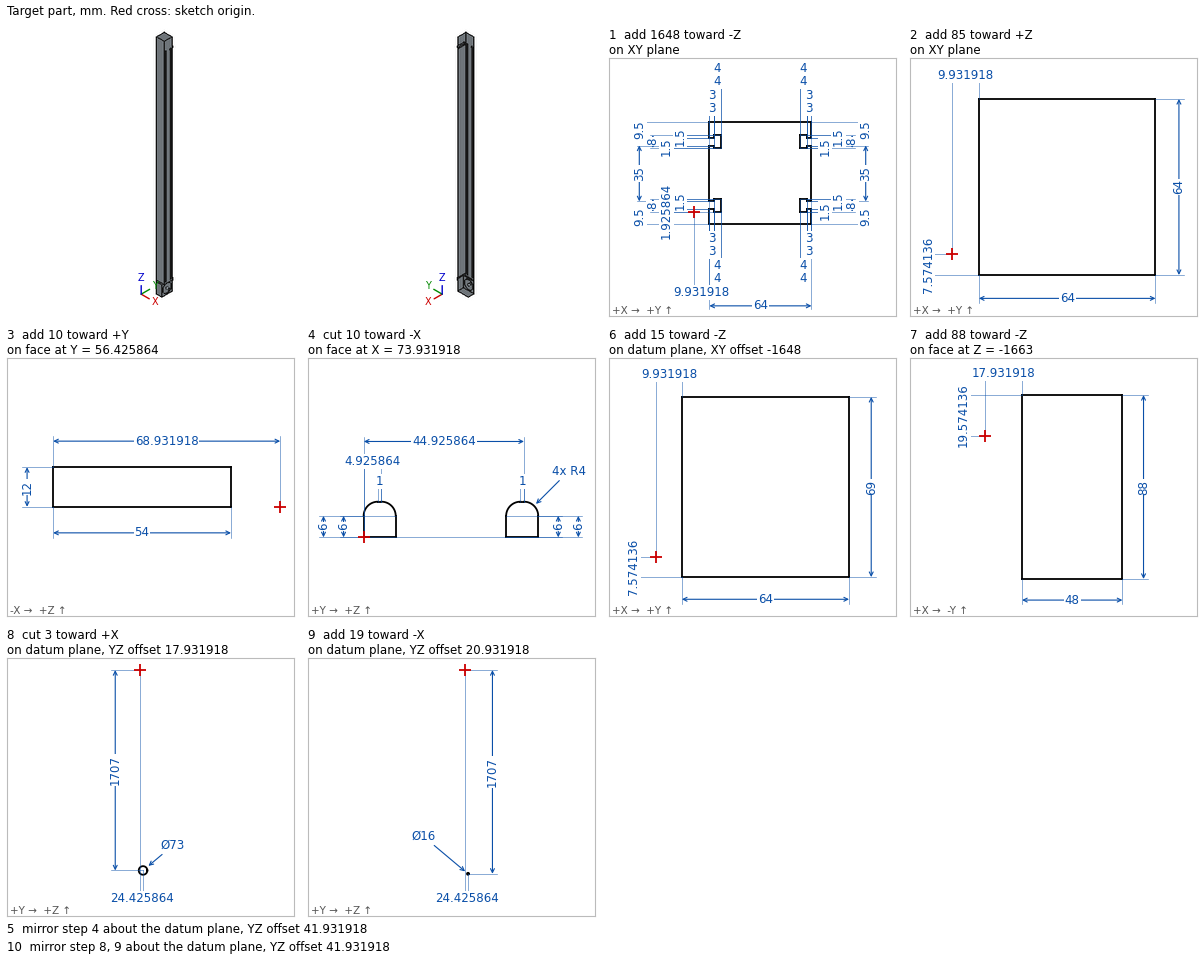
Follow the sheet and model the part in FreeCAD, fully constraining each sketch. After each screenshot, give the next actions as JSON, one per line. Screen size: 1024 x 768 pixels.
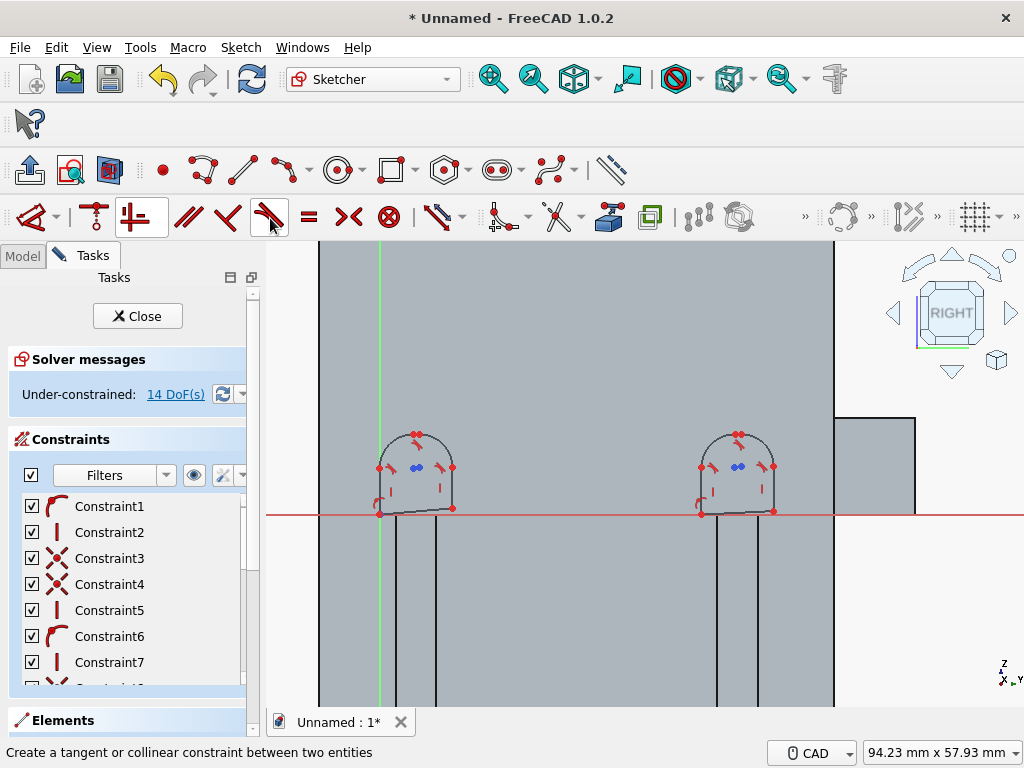
{"action": "left_click", "coordinate": [723, 514]}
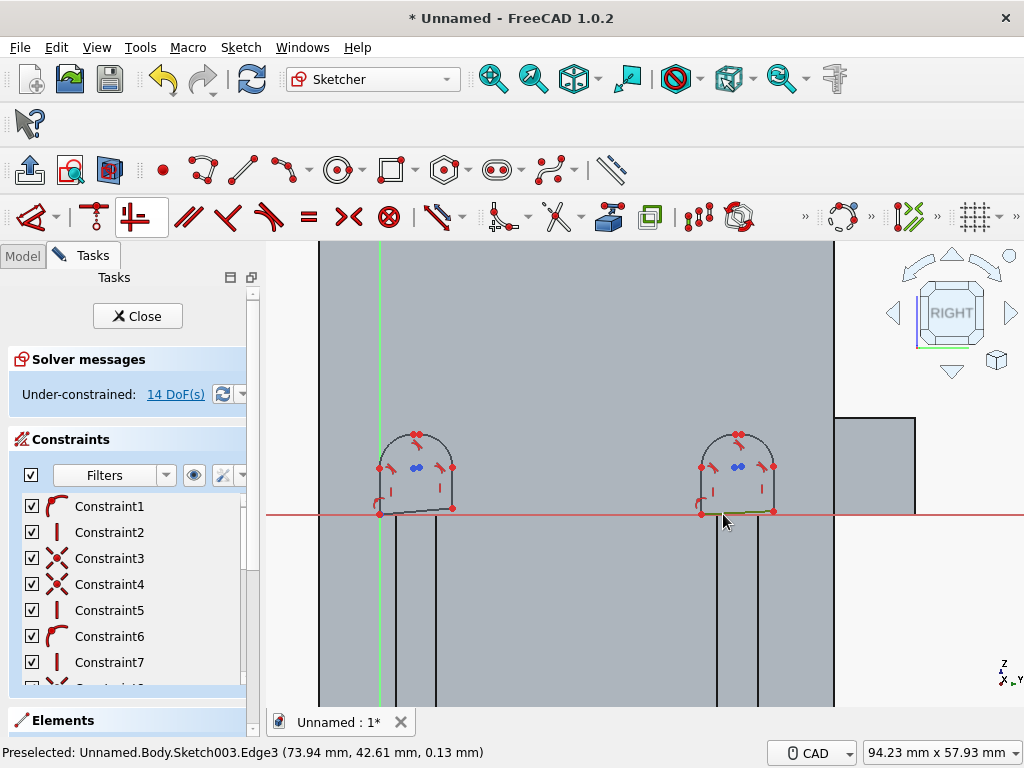
{"action": "left_click", "coordinate": [162, 218]}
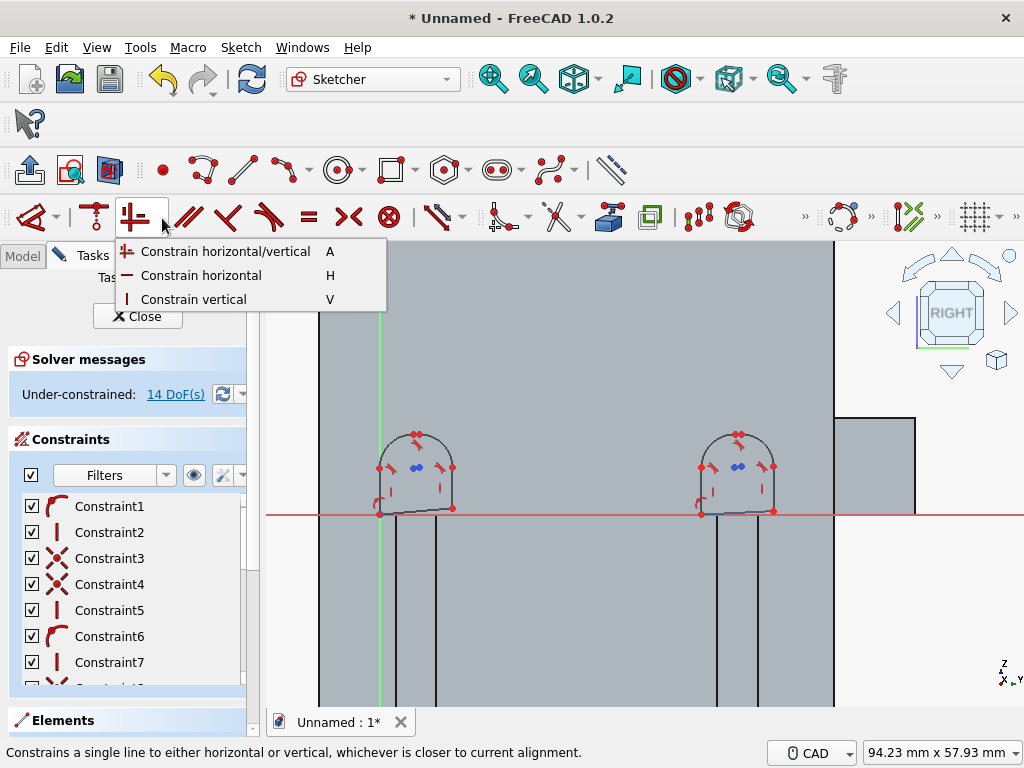
{"action": "left_click", "coordinate": [251, 275]}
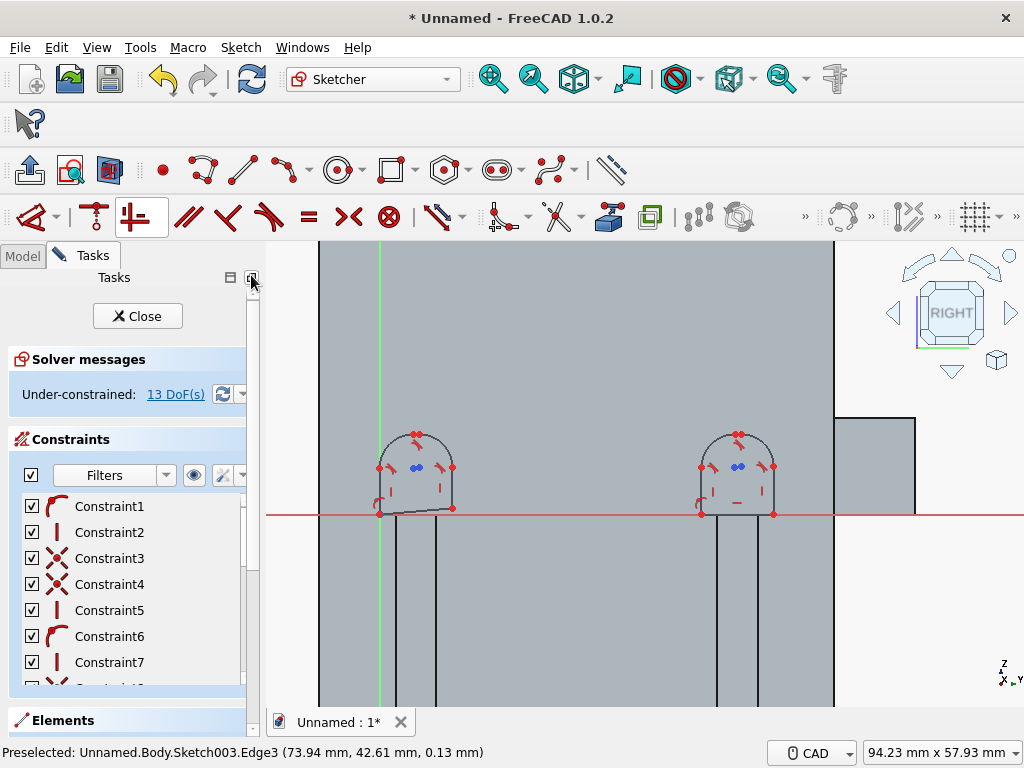
{"action": "left_click", "coordinate": [402, 513]}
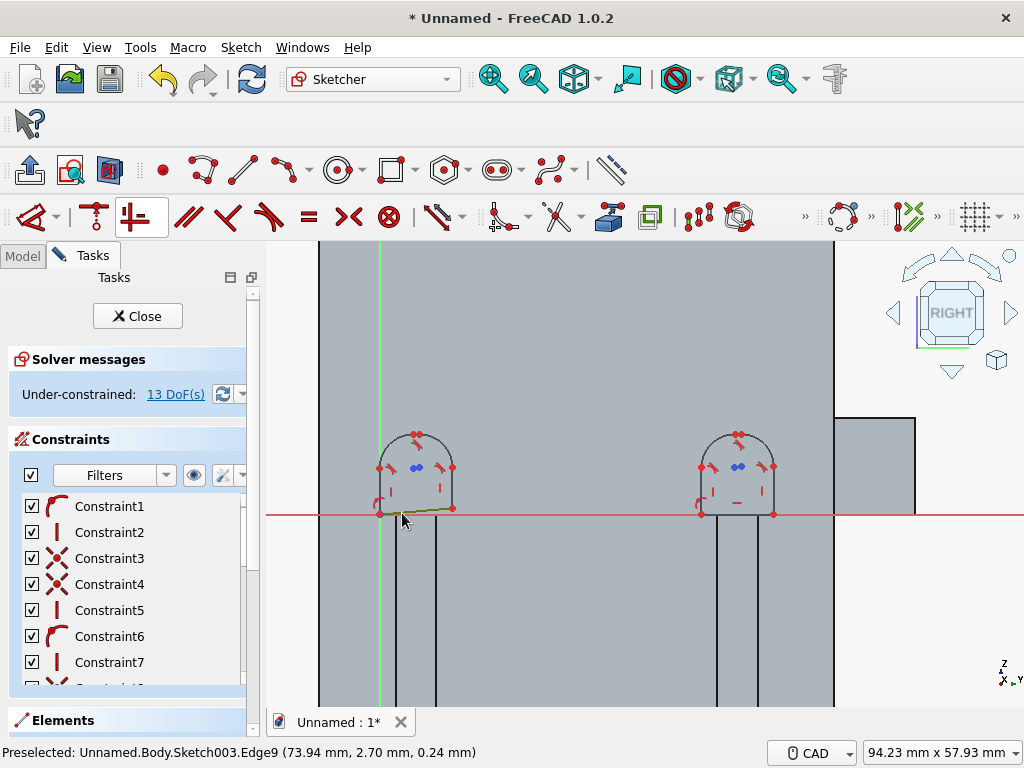
{"action": "key", "text": "h"}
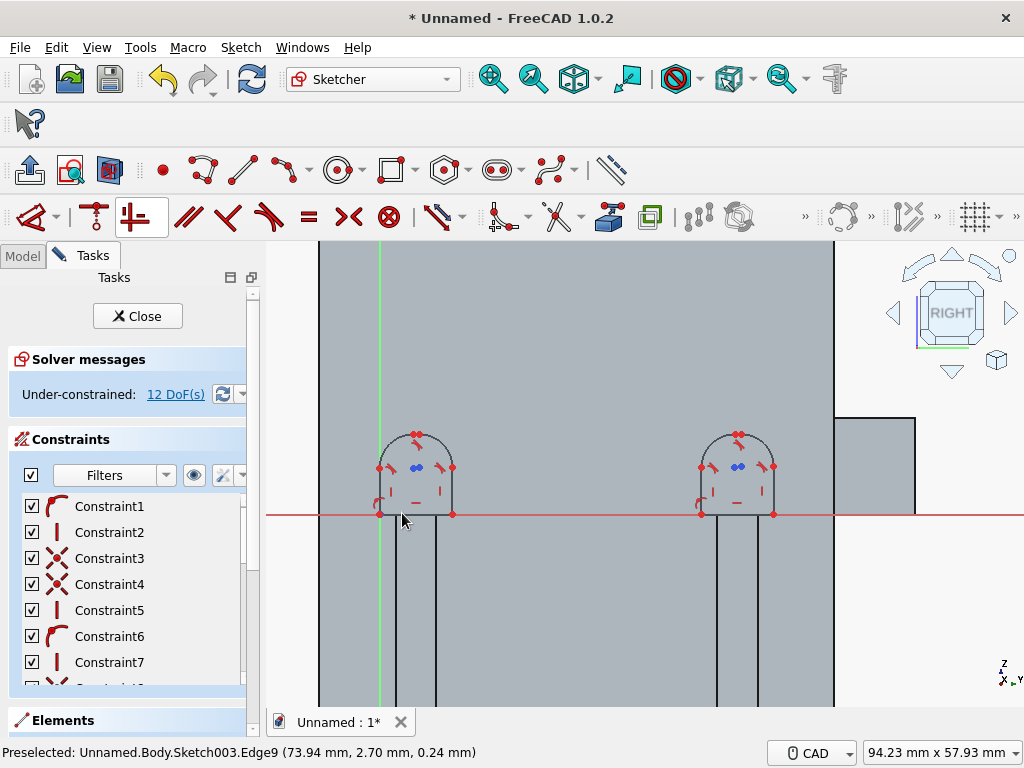
{"action": "left_click", "coordinate": [720, 438]}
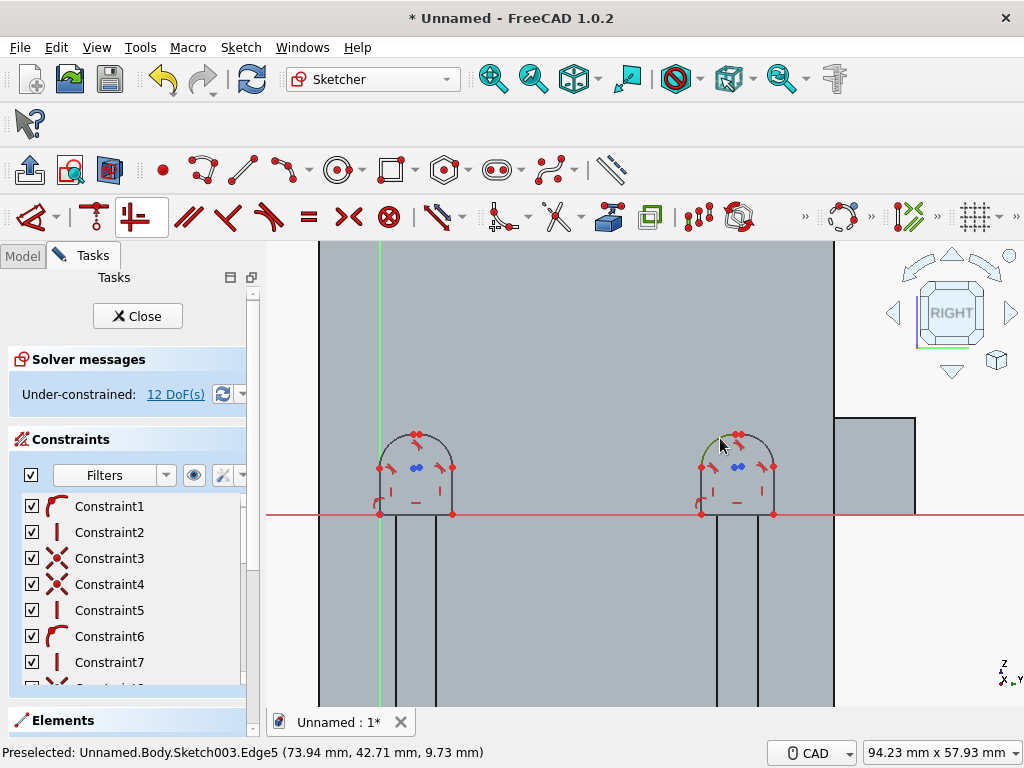
{"action": "left_click", "coordinate": [770, 452]}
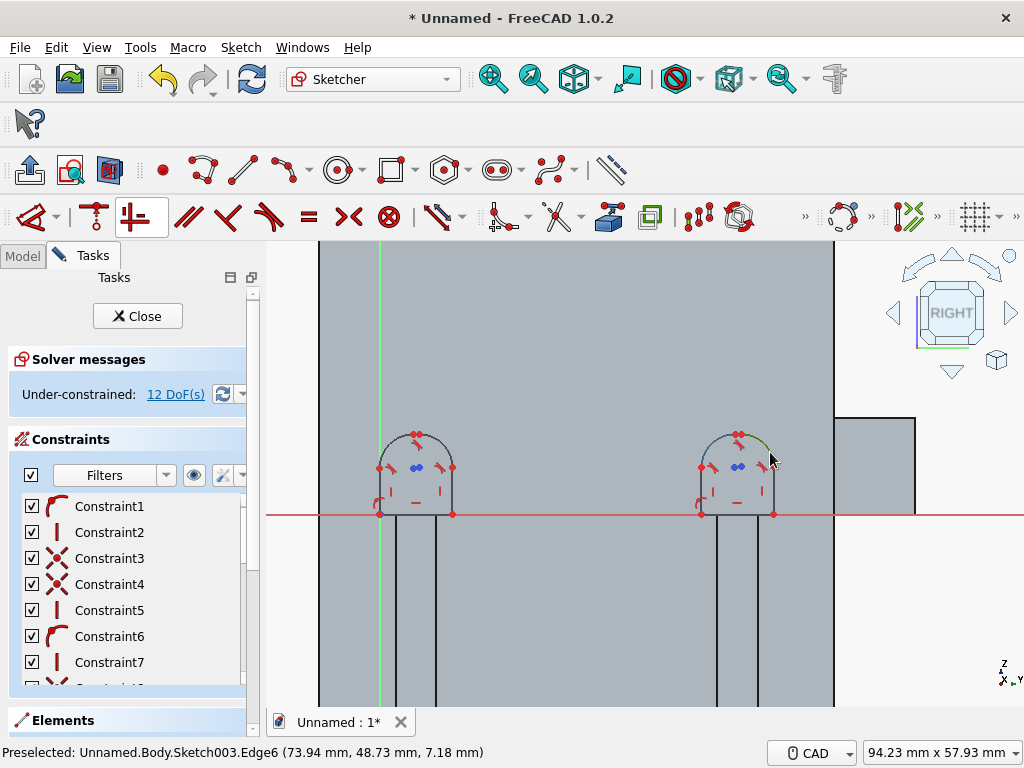
{"action": "left_click", "coordinate": [398, 438]}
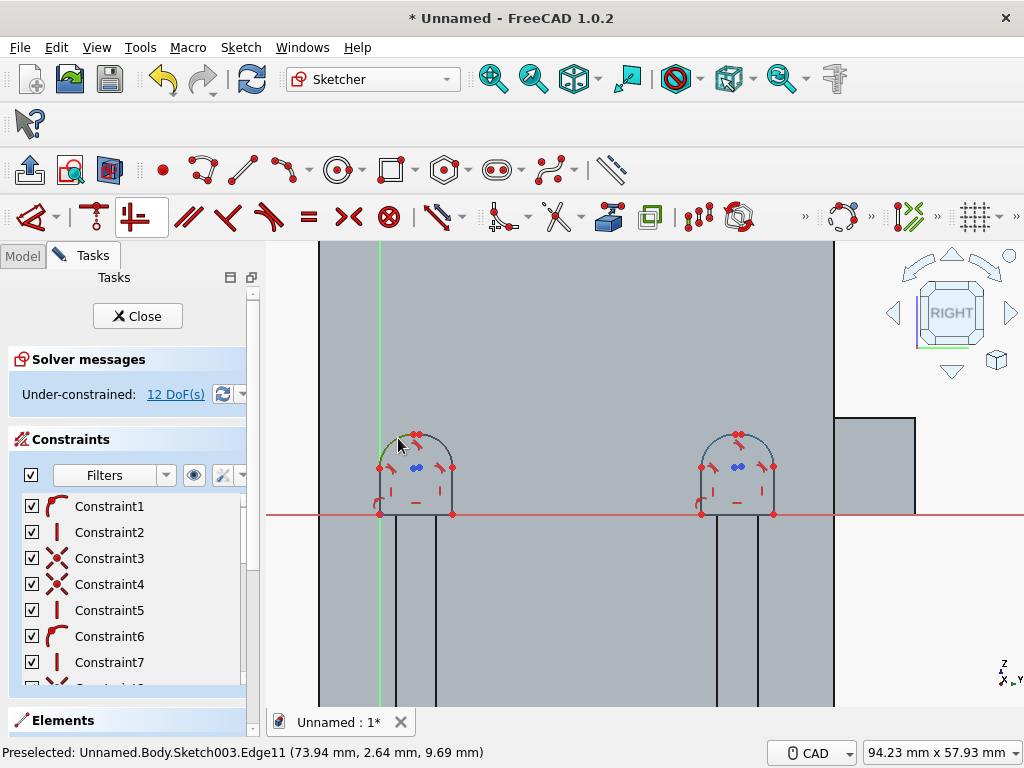
{"action": "left_click", "coordinate": [449, 453]}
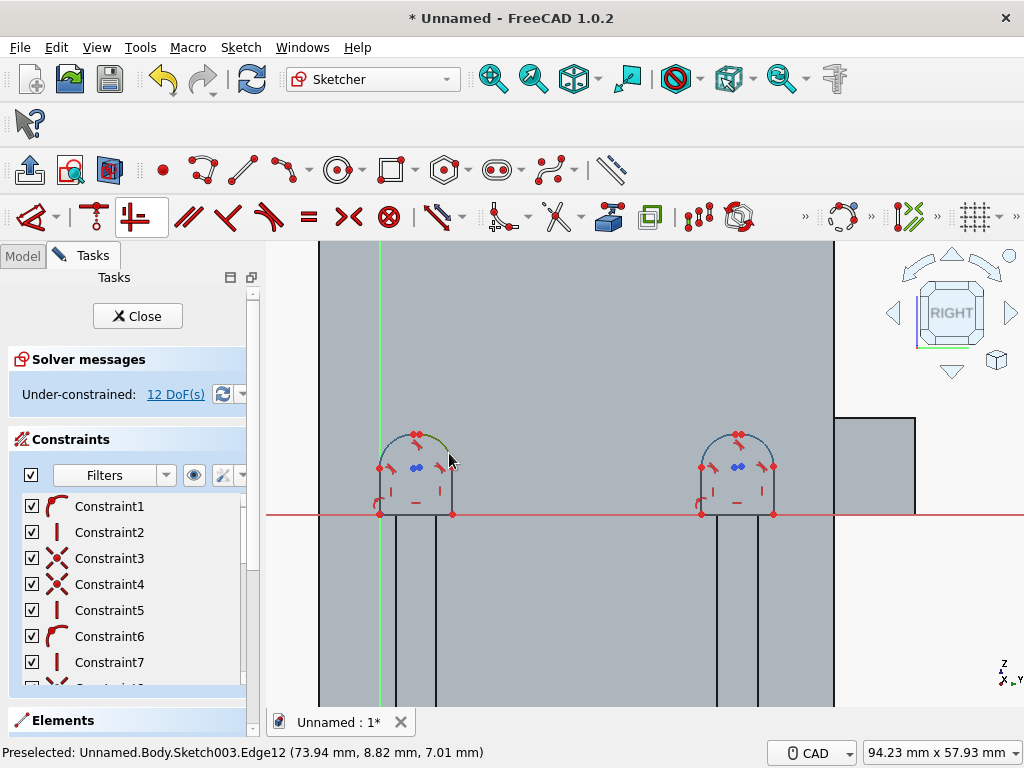
{"action": "left_click", "coordinate": [310, 218]}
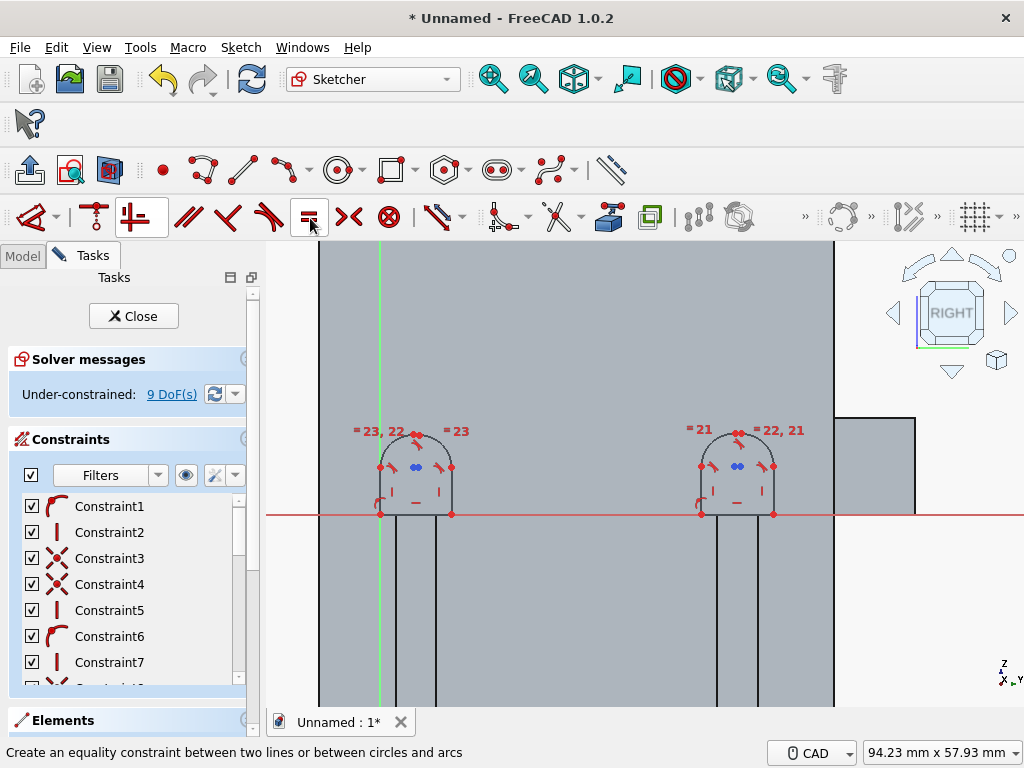
{"action": "left_click", "coordinate": [32, 218]}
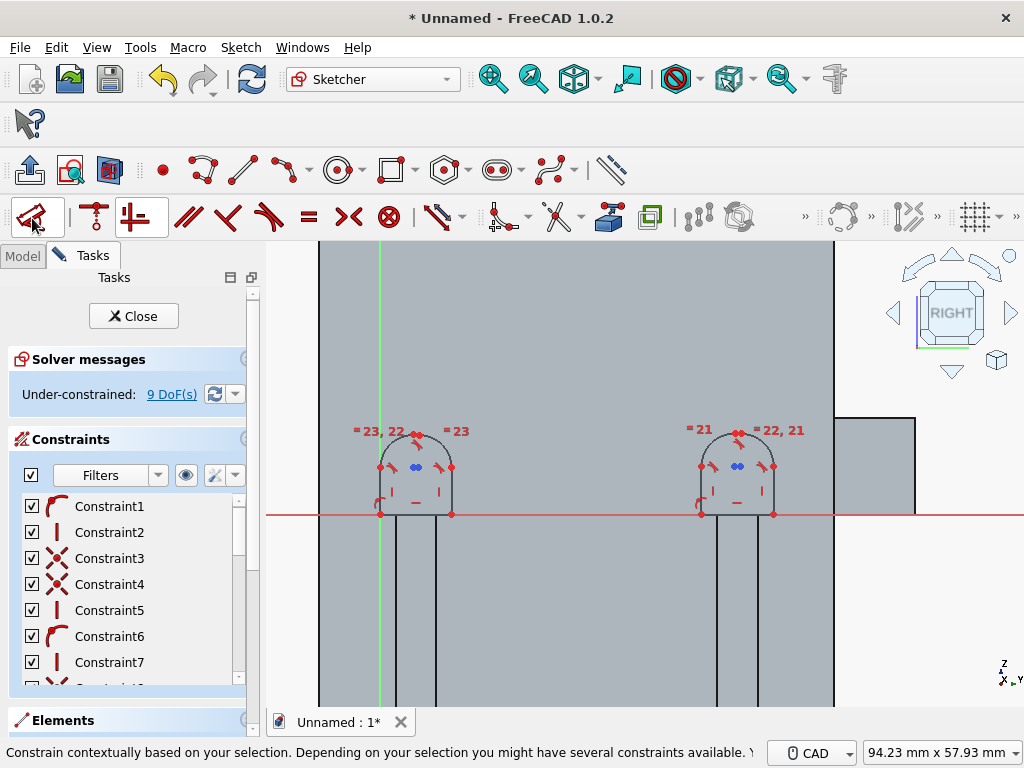
{"action": "scroll", "coordinate": [720, 437], "scroll_direction": "up", "scroll_amount": 2}